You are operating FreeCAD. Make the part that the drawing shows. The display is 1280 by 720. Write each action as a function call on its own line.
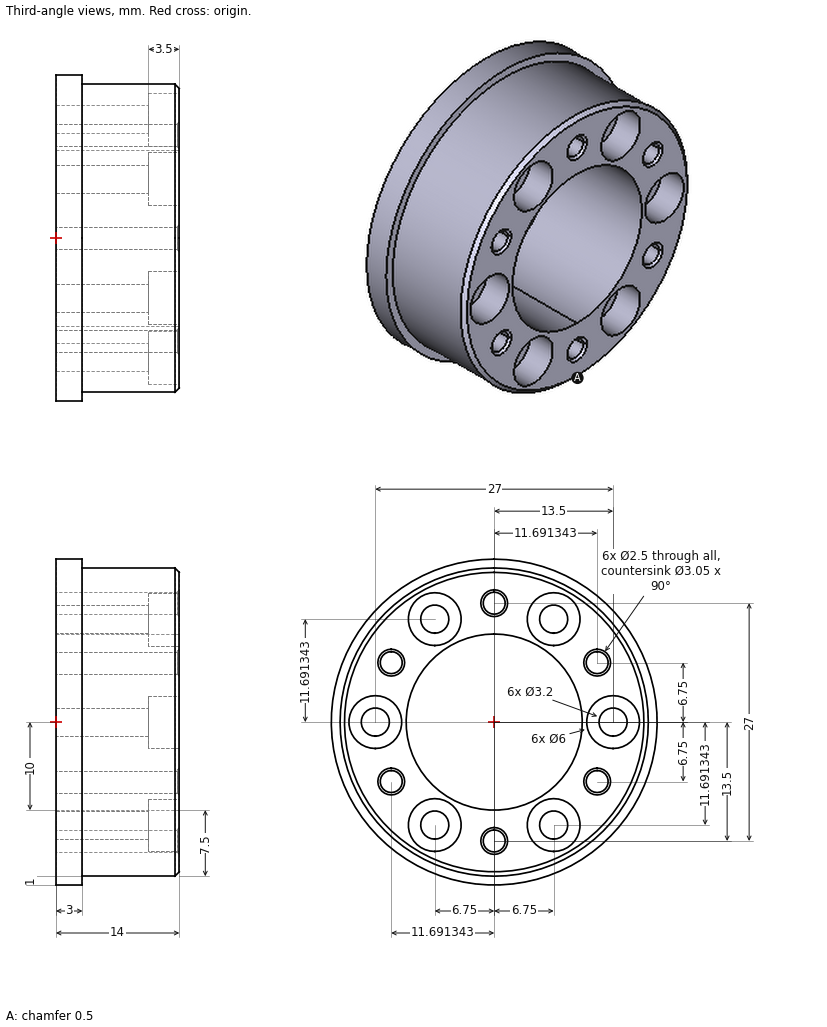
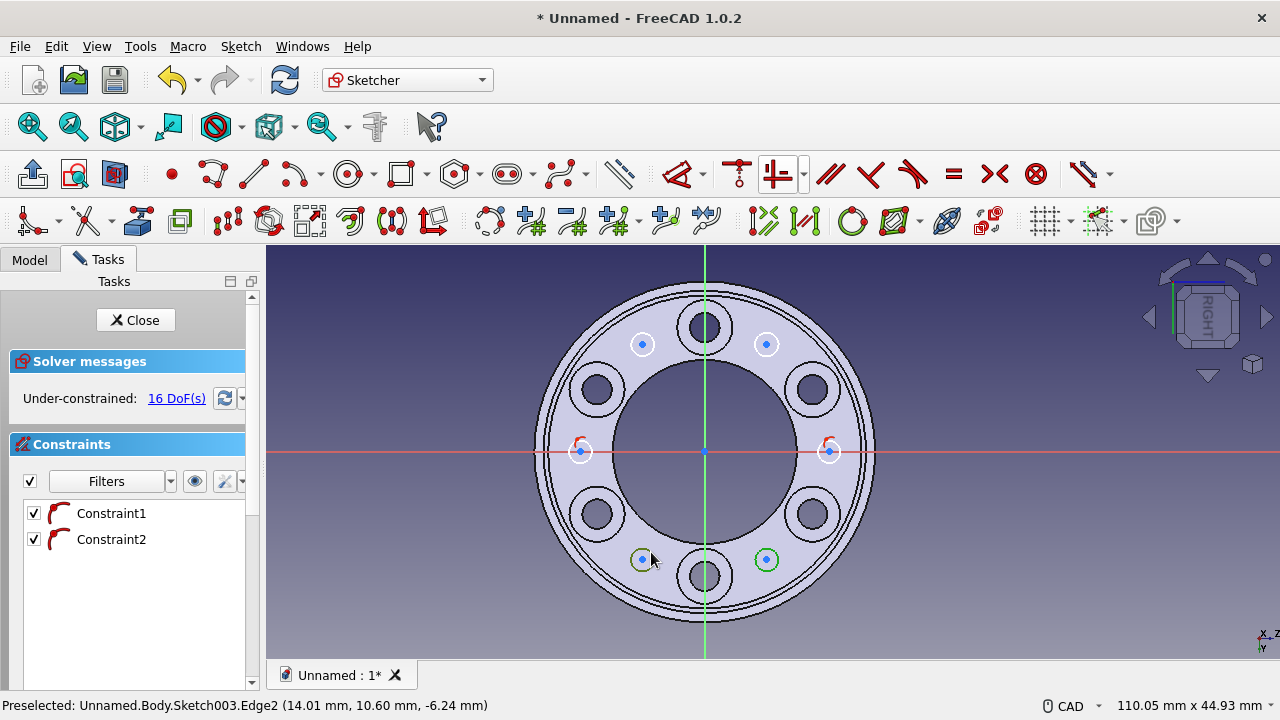
scroll(581, 441, up, 2)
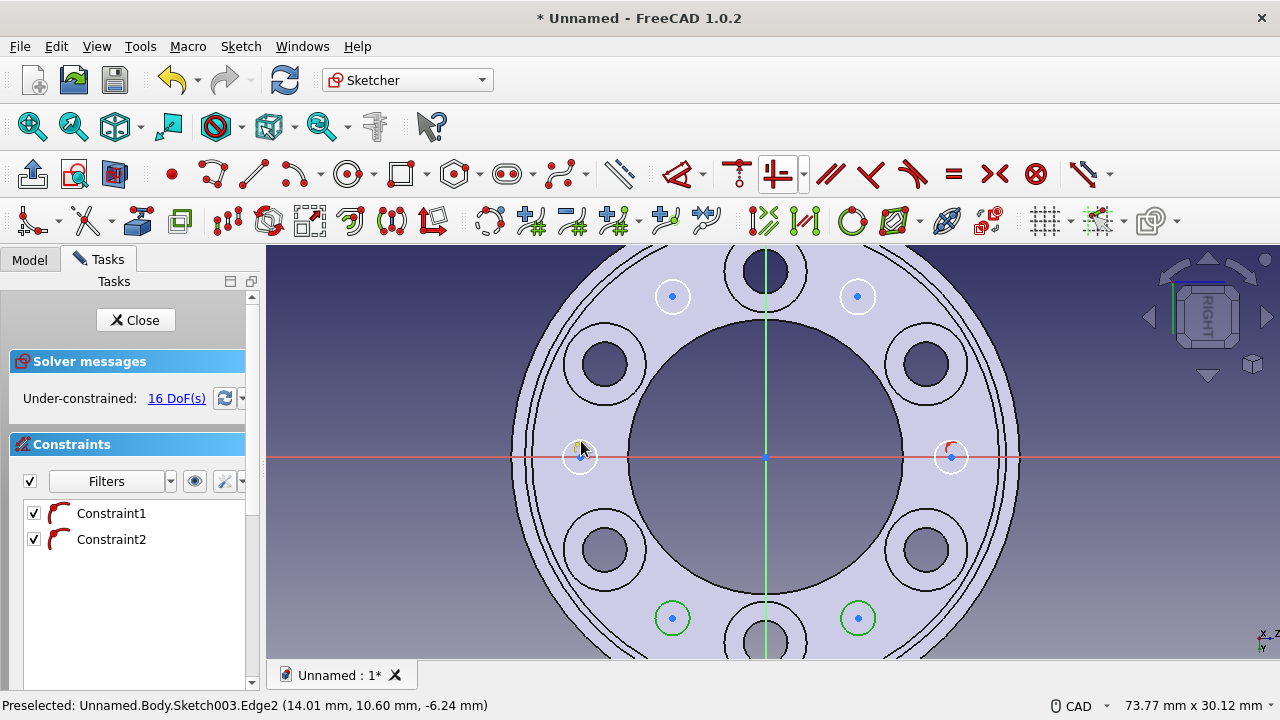
click(563, 457)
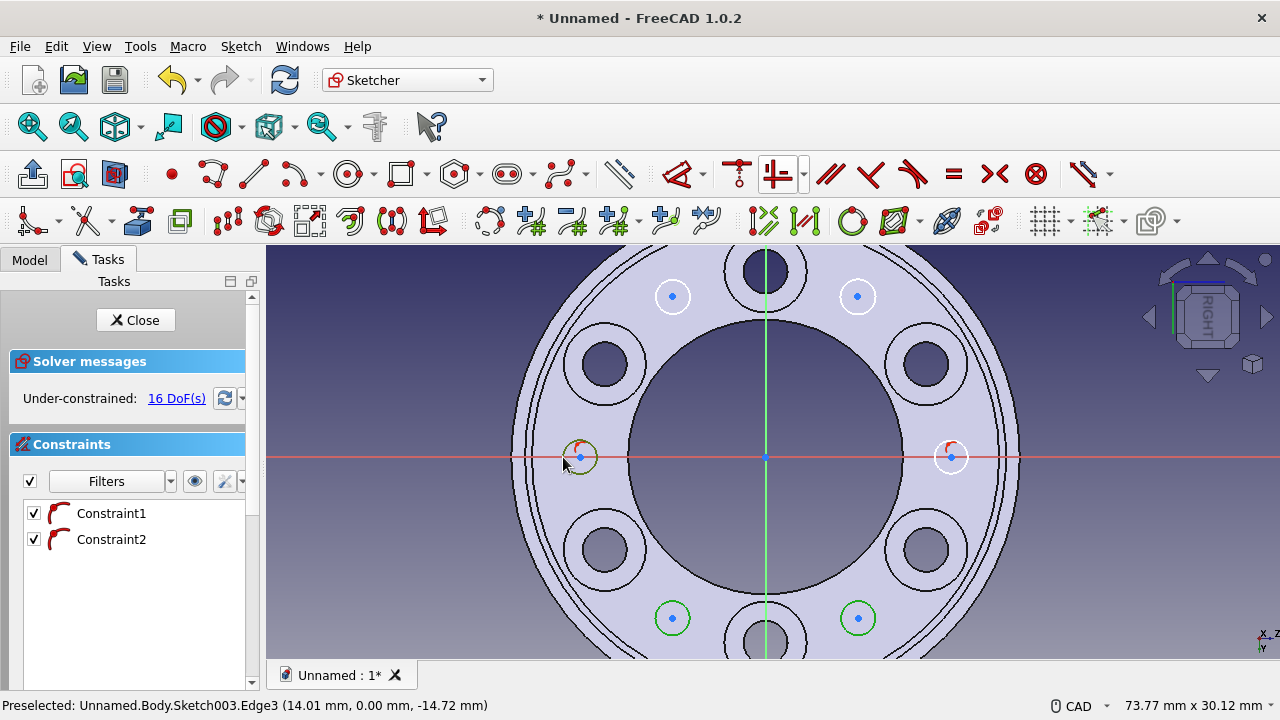
click(685, 285)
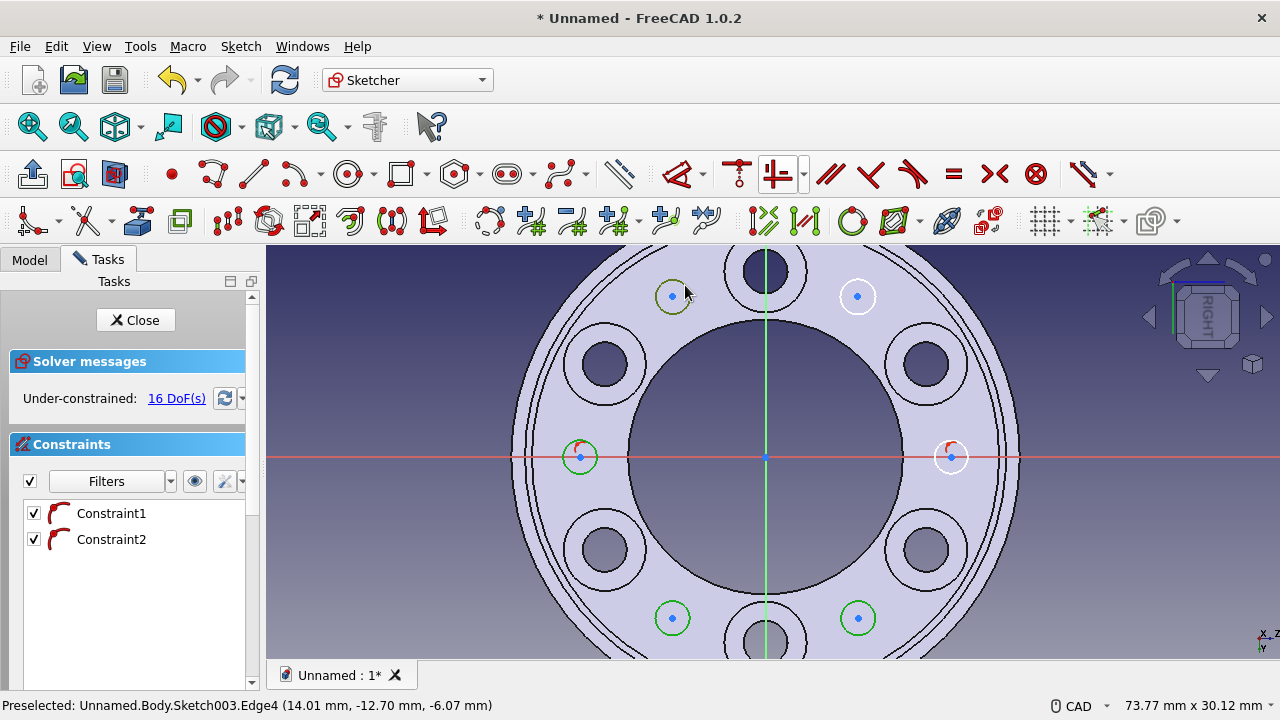
click(870, 284)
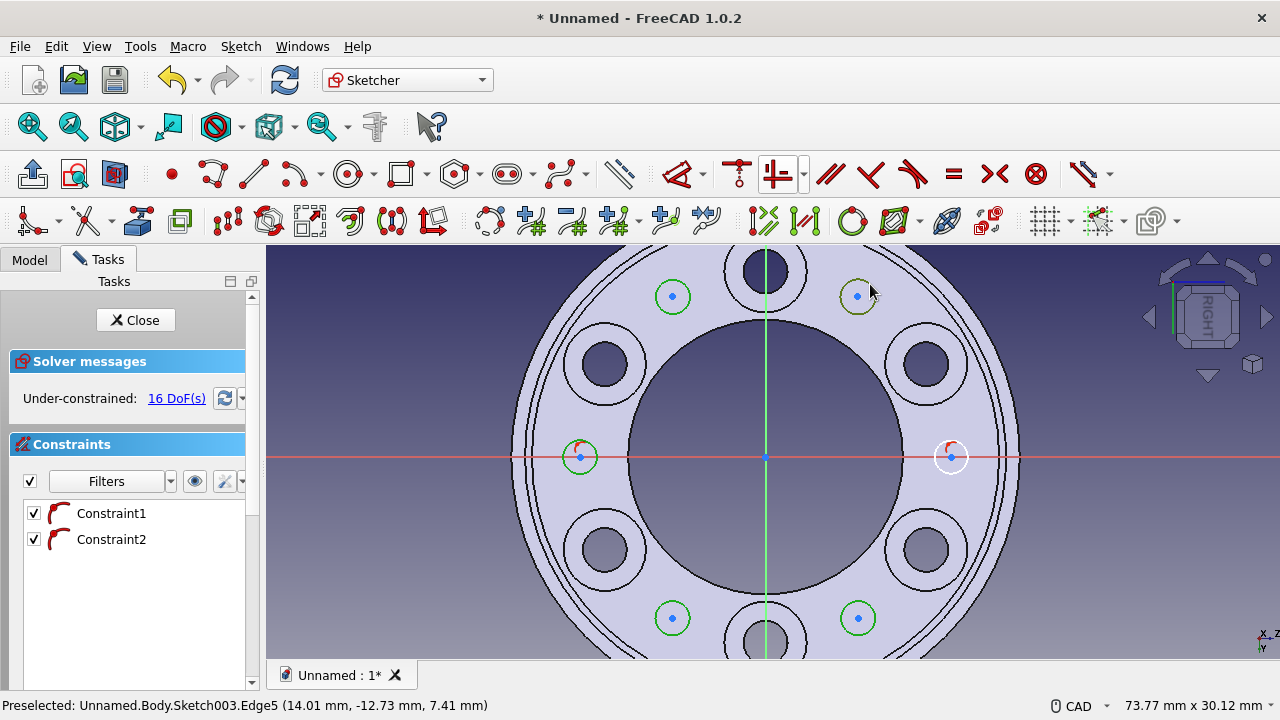
click(963, 445)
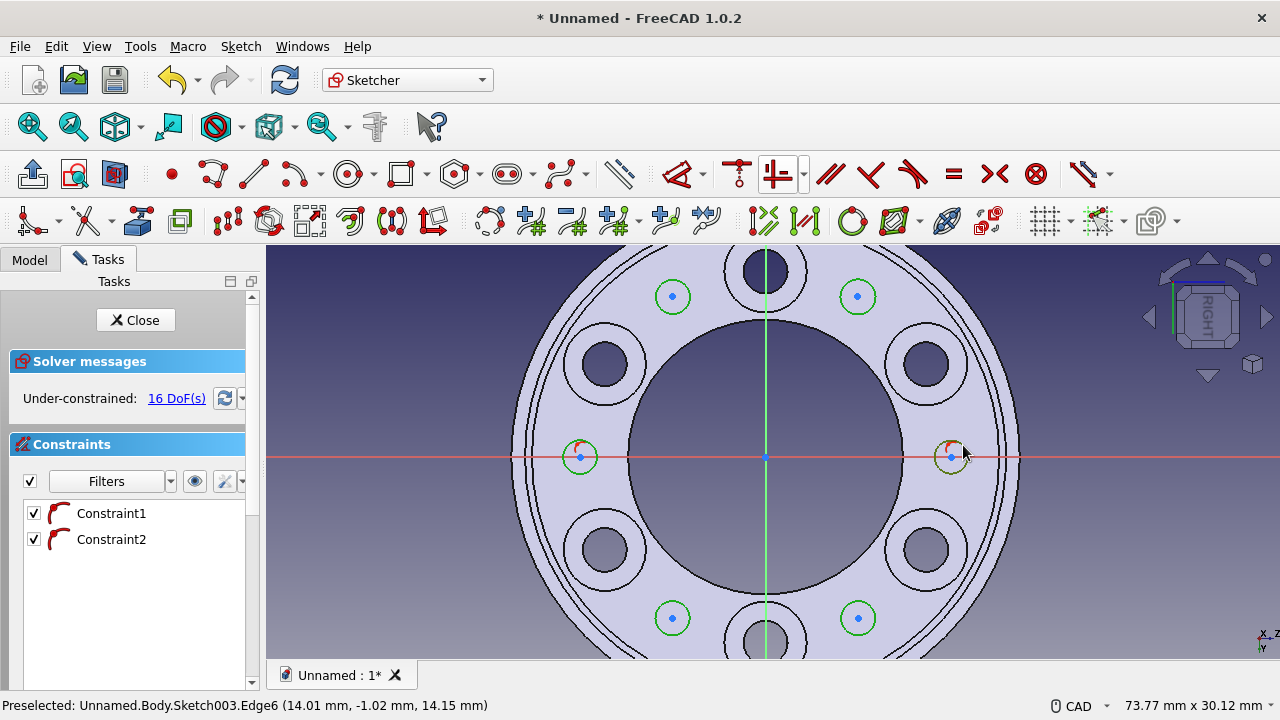
click(954, 174)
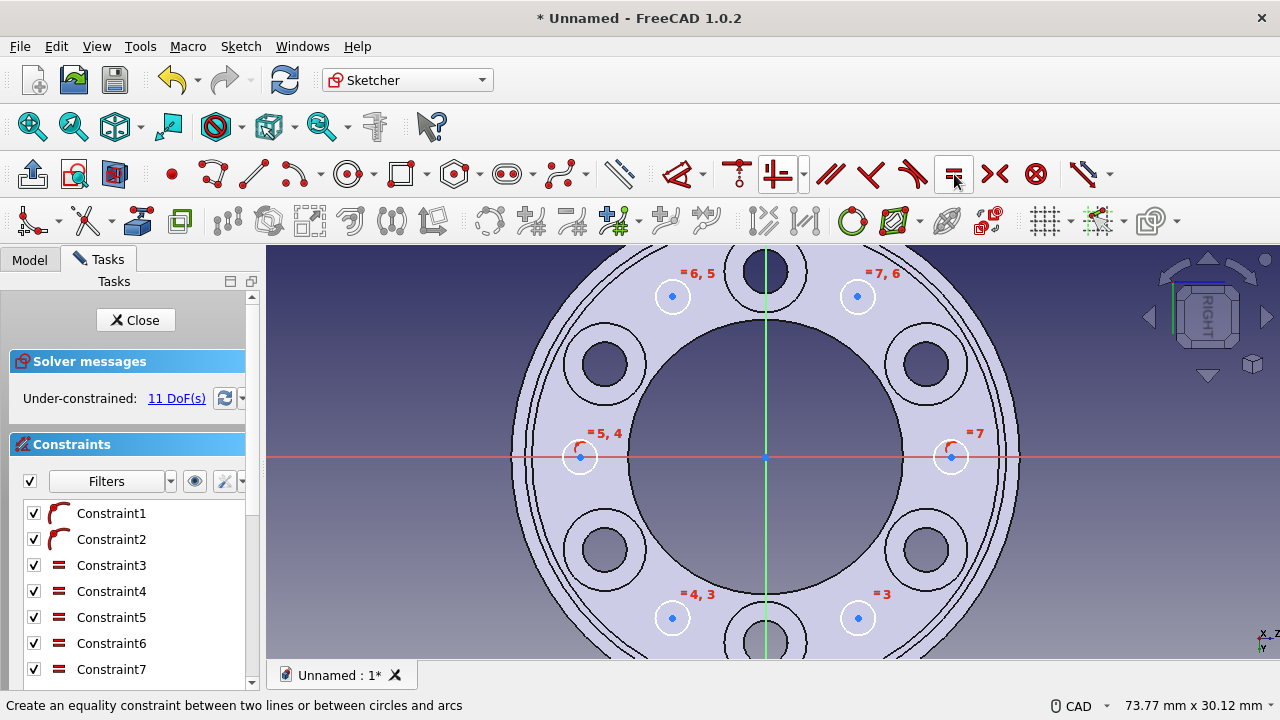
click(858, 618)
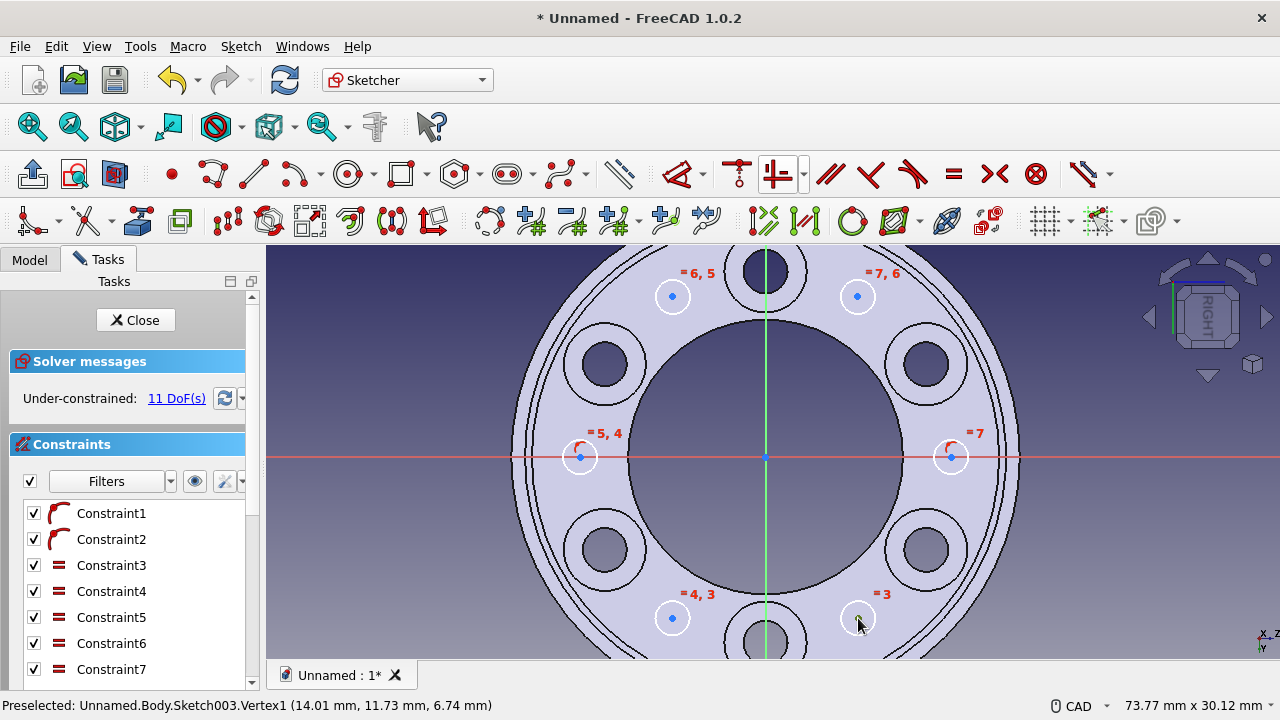
click(673, 618)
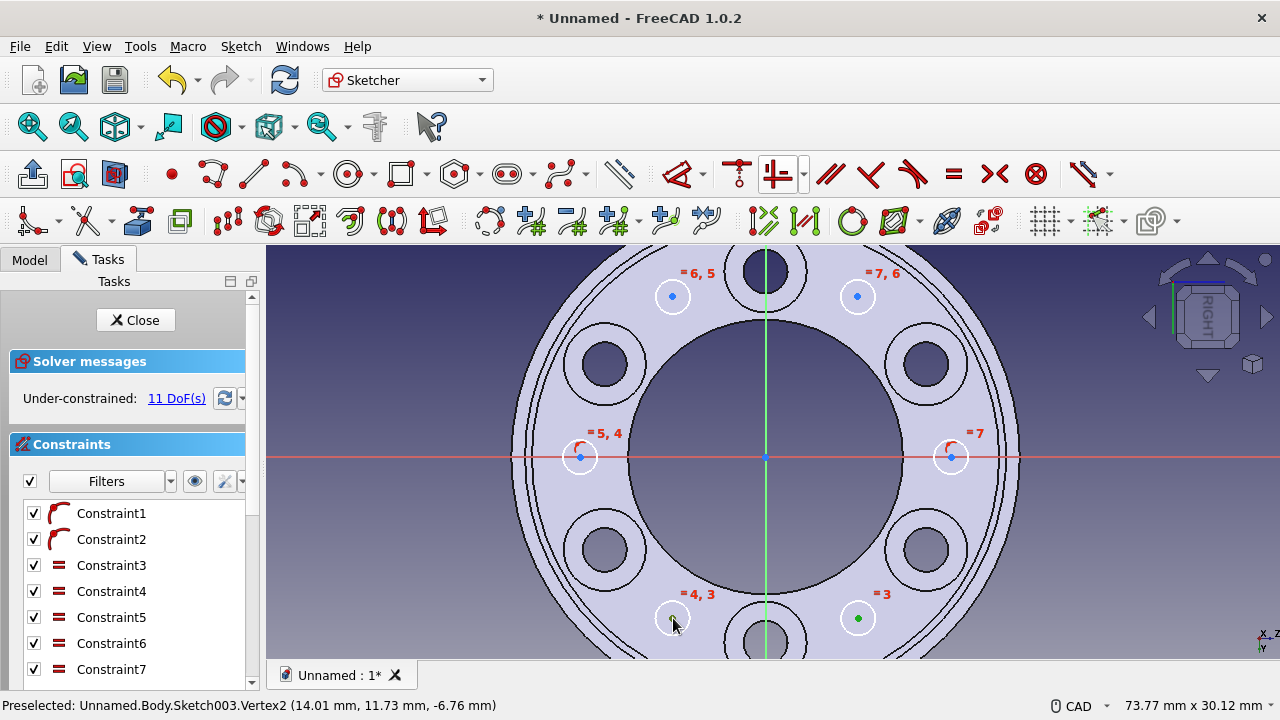
key(h)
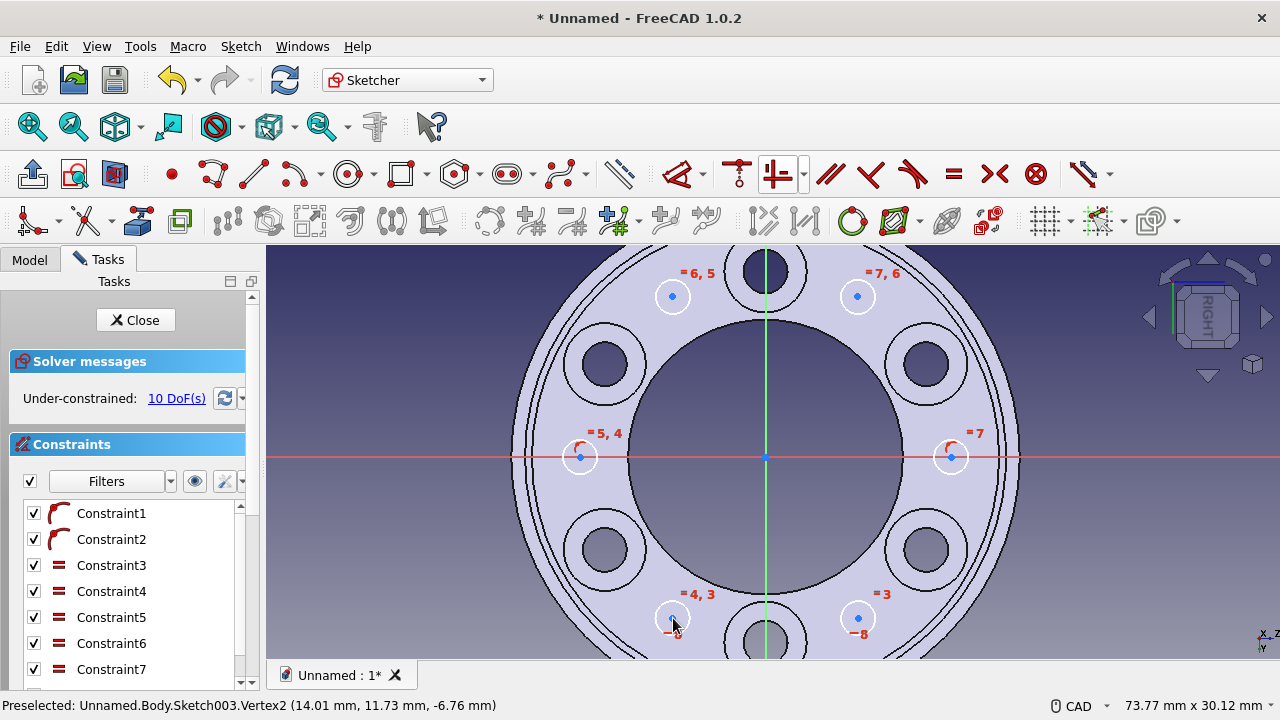
click(673, 618)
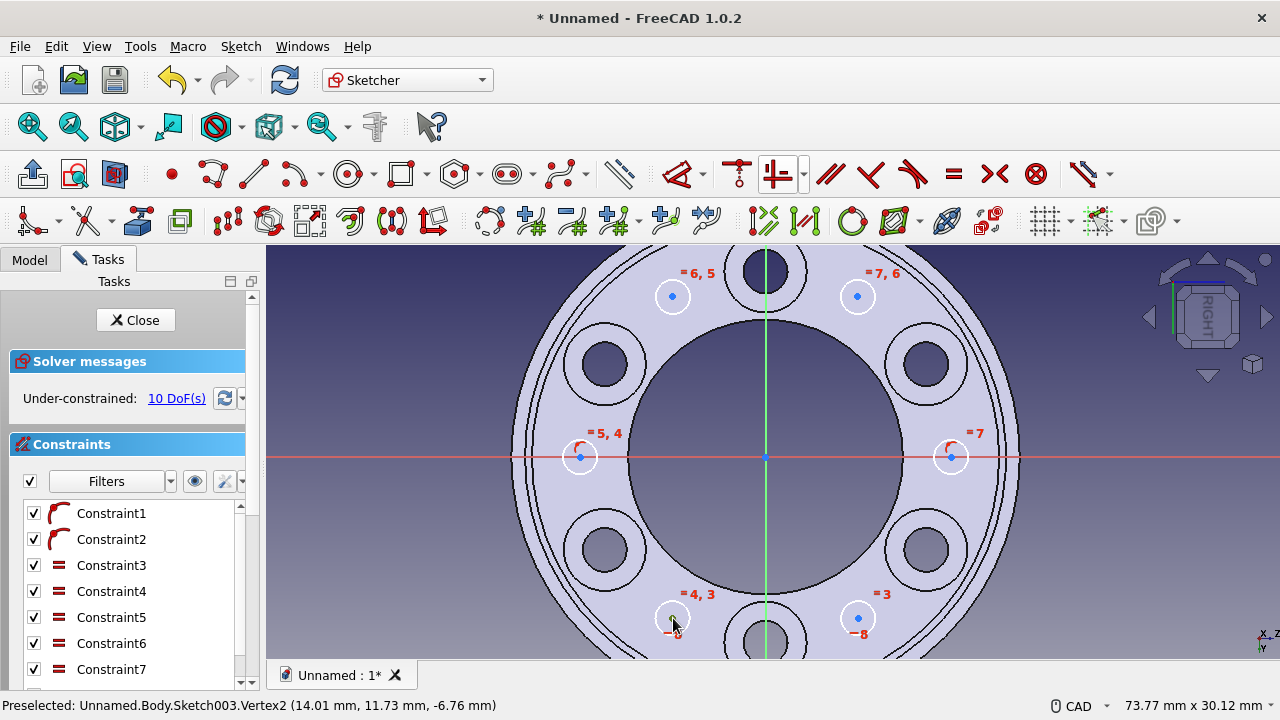
click(673, 297)